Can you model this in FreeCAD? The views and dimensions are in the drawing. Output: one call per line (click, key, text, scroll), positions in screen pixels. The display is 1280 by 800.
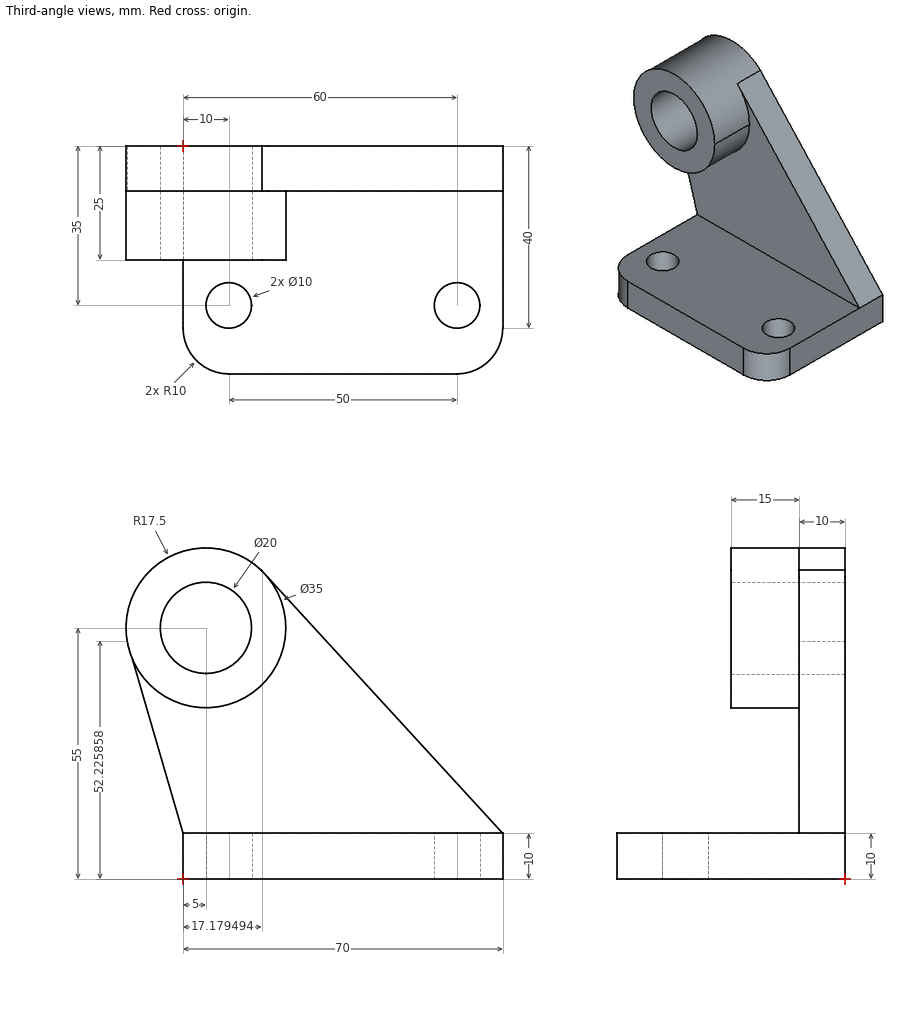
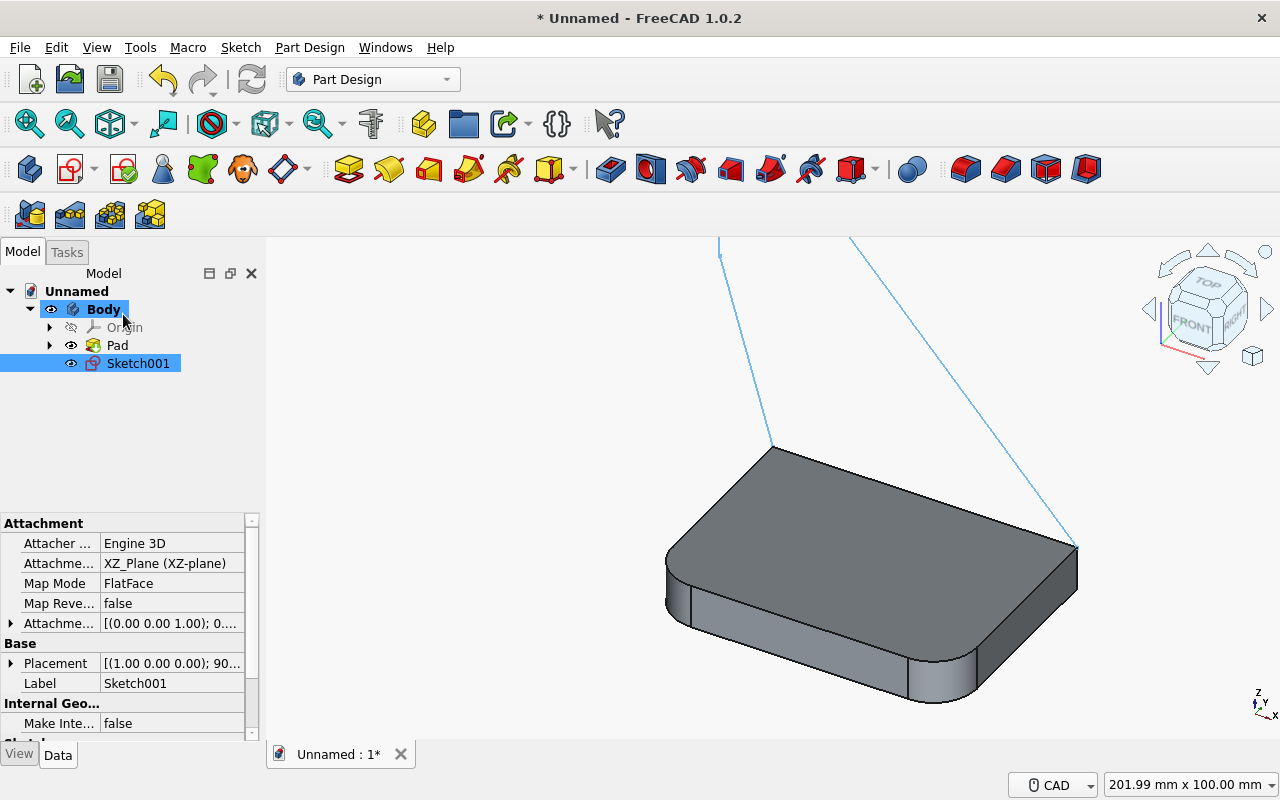
click(350, 170)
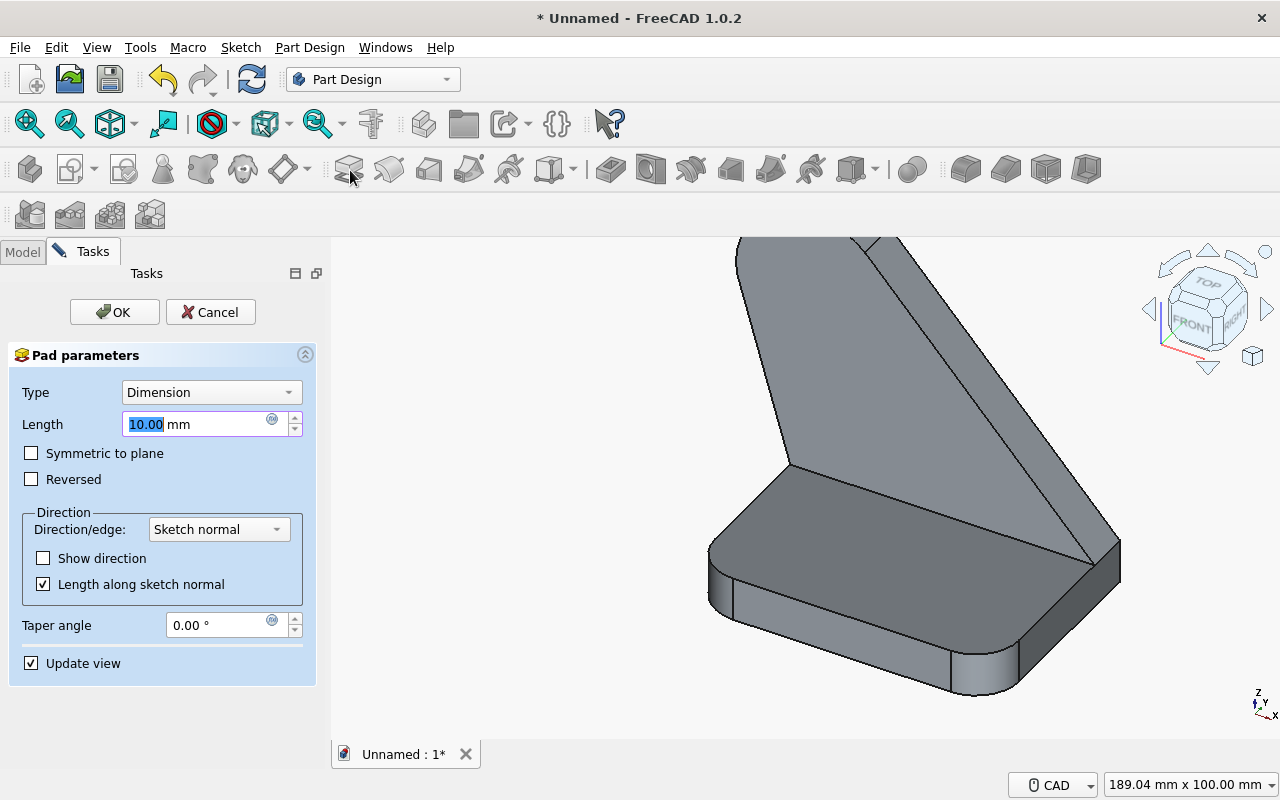
text(10)
key(Tab)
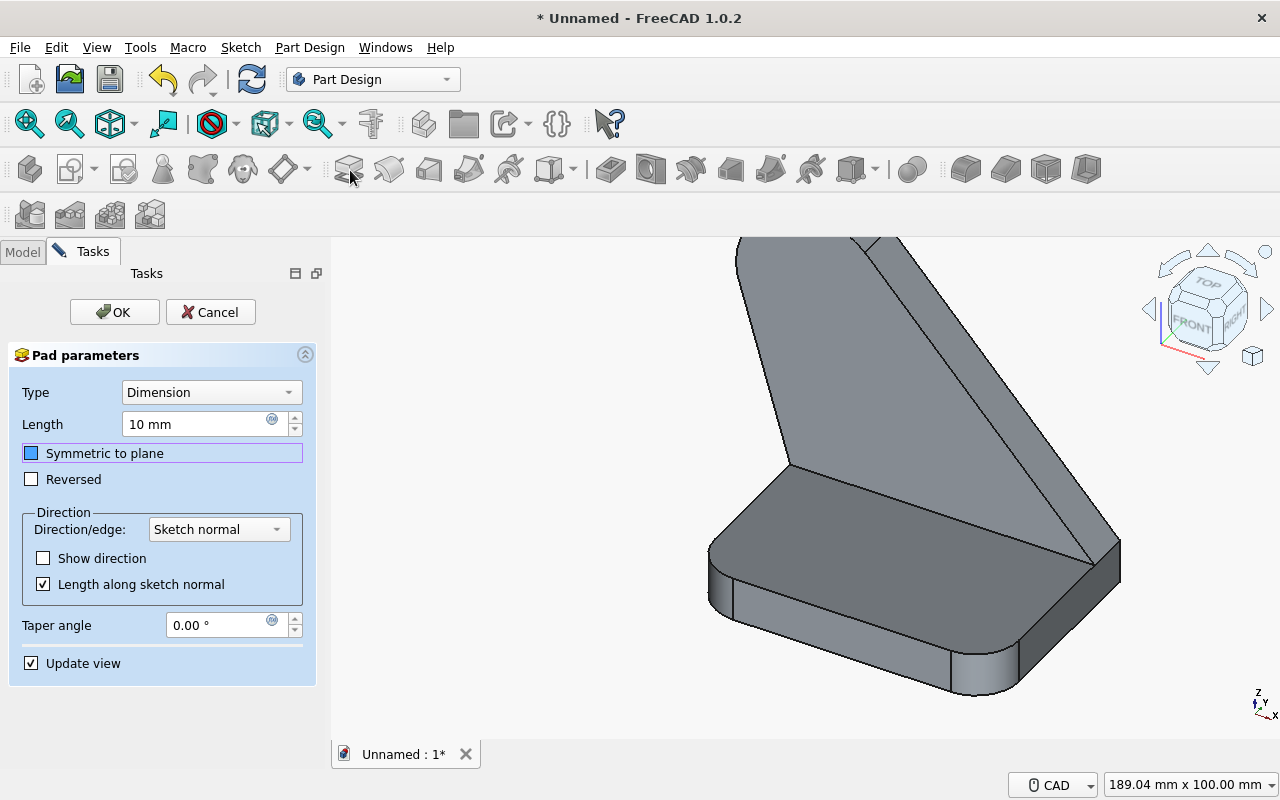
click(115, 312)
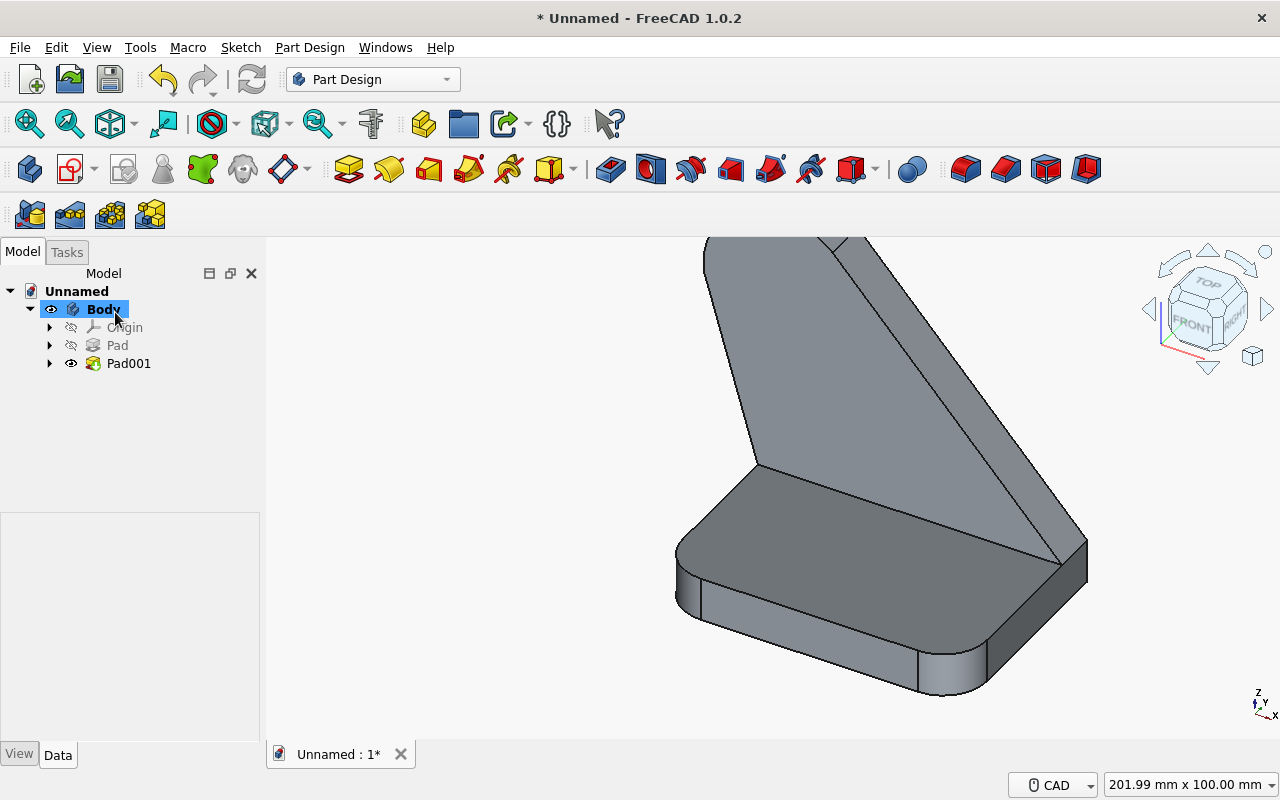
key(v)
key(f)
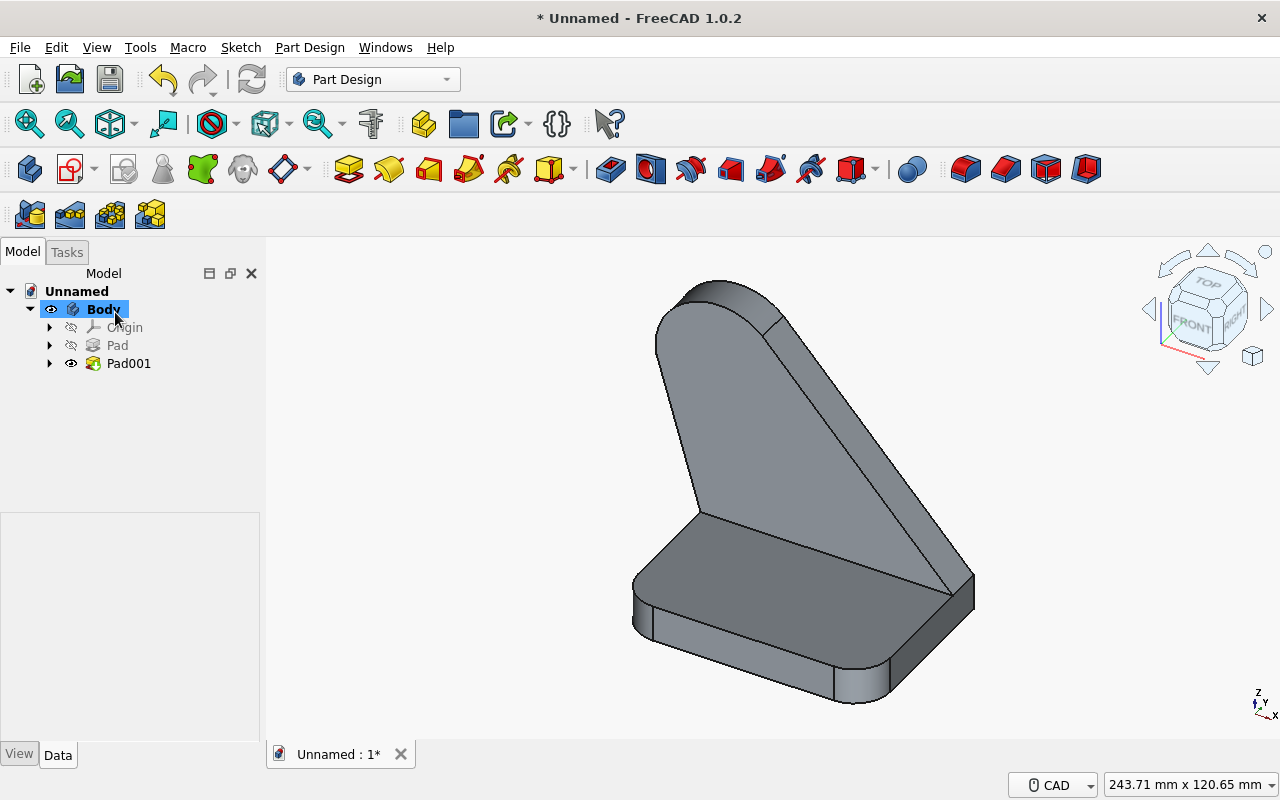
click(762, 455)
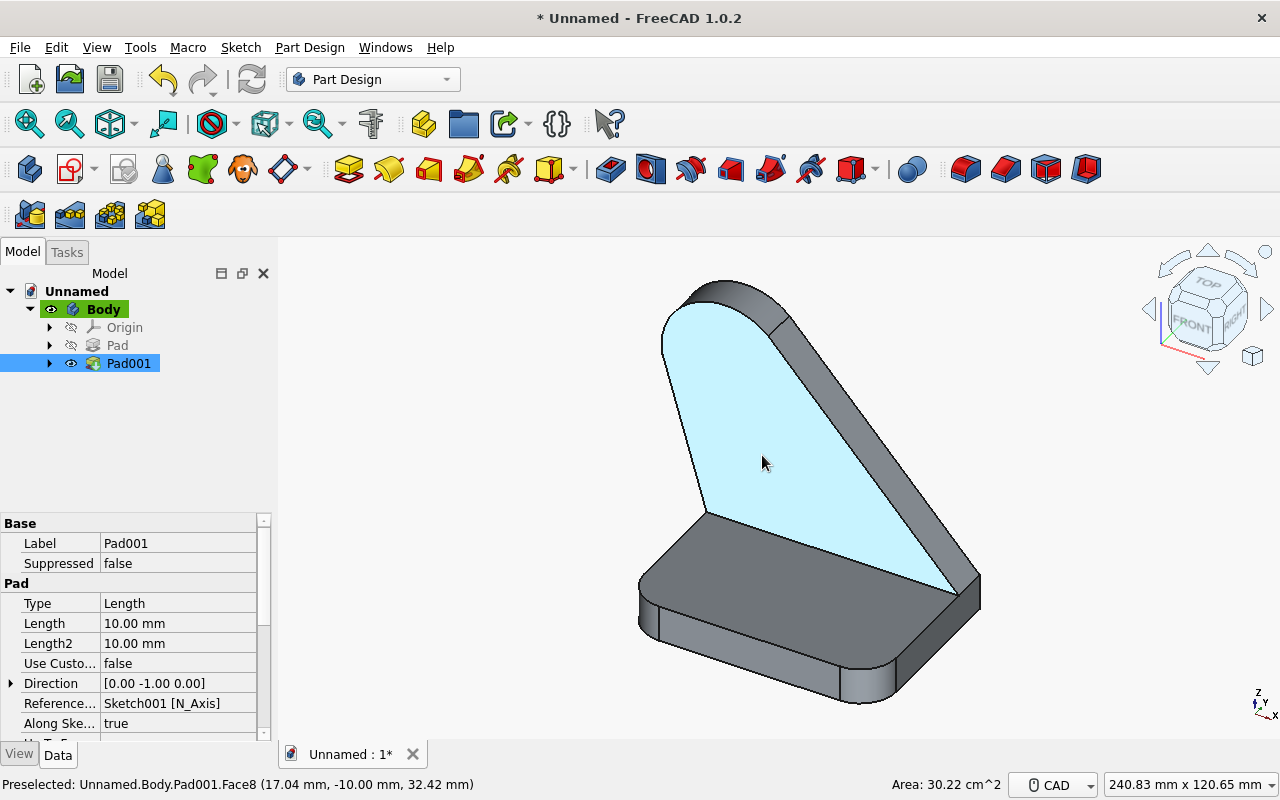
click(70, 170)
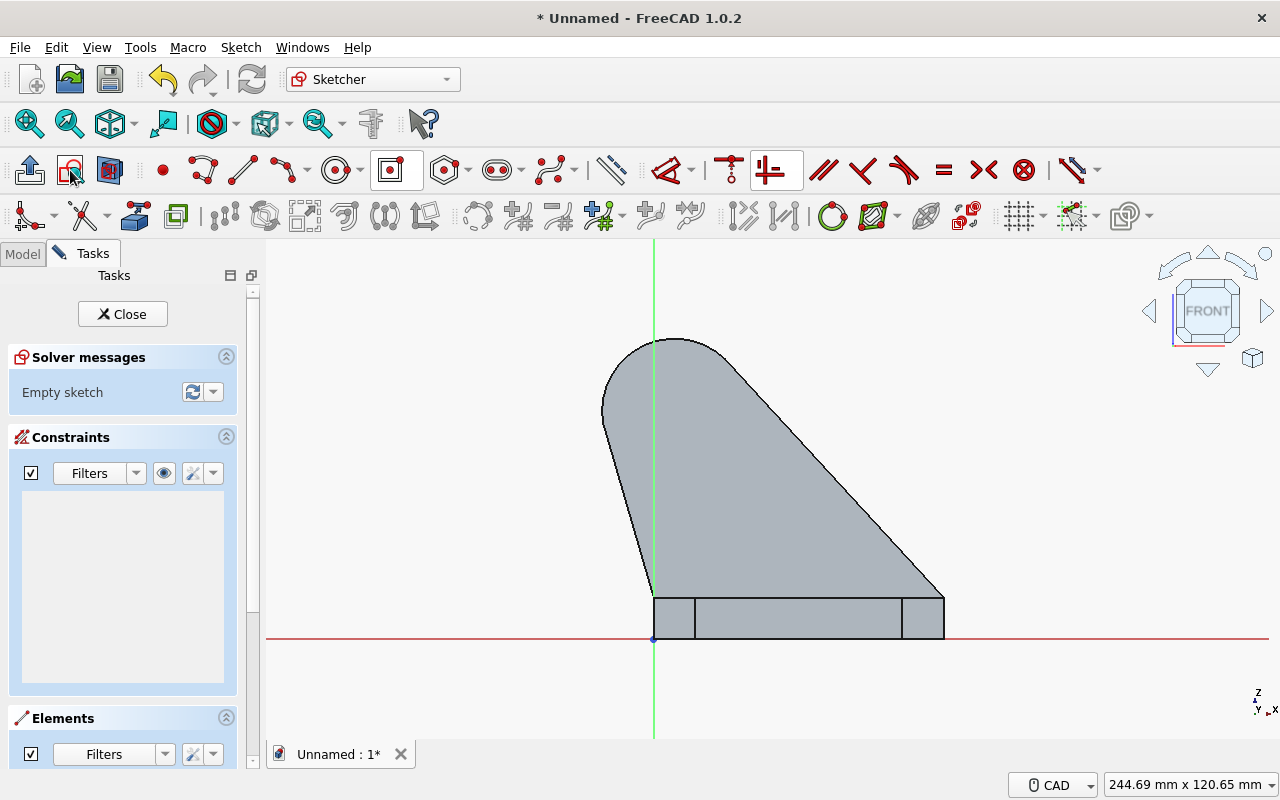
key(q)
key(s)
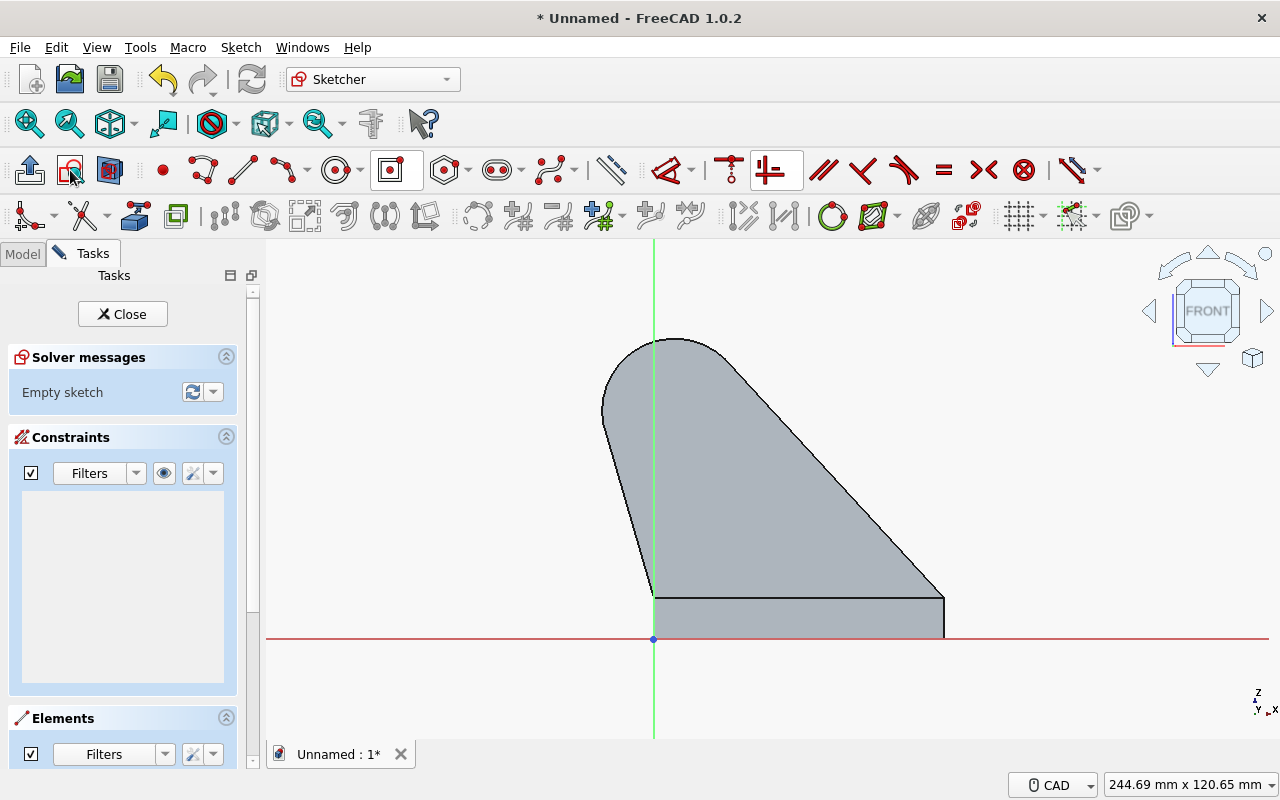
click(336, 170)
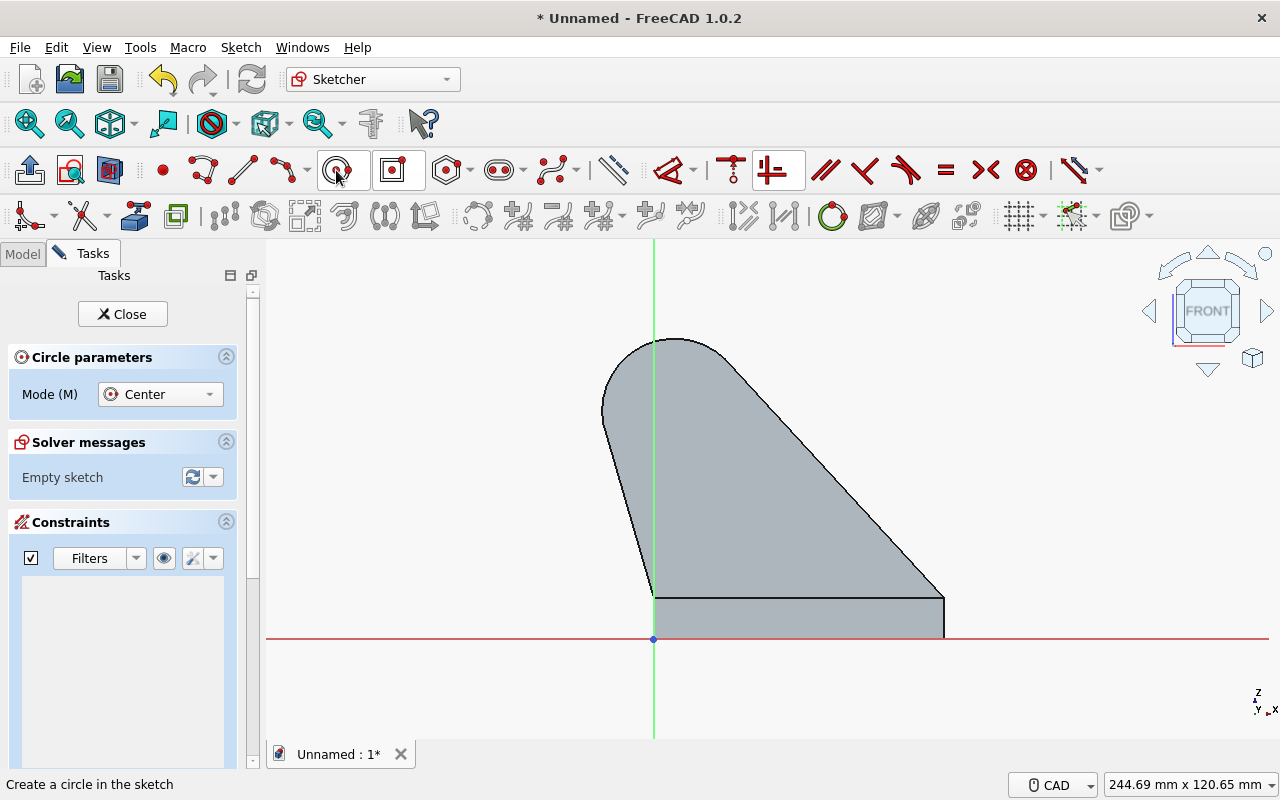
click(675, 411)
click(726, 360)
key(Escape)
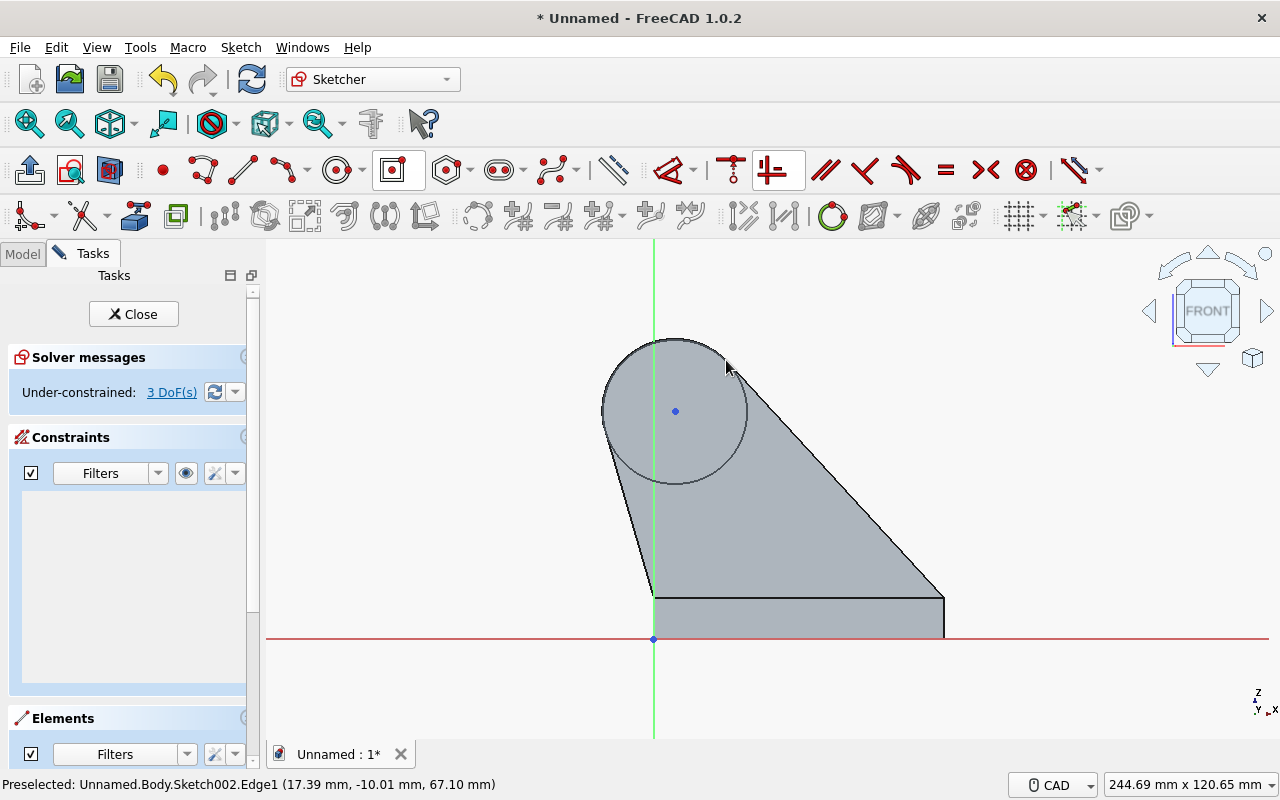
click(668, 170)